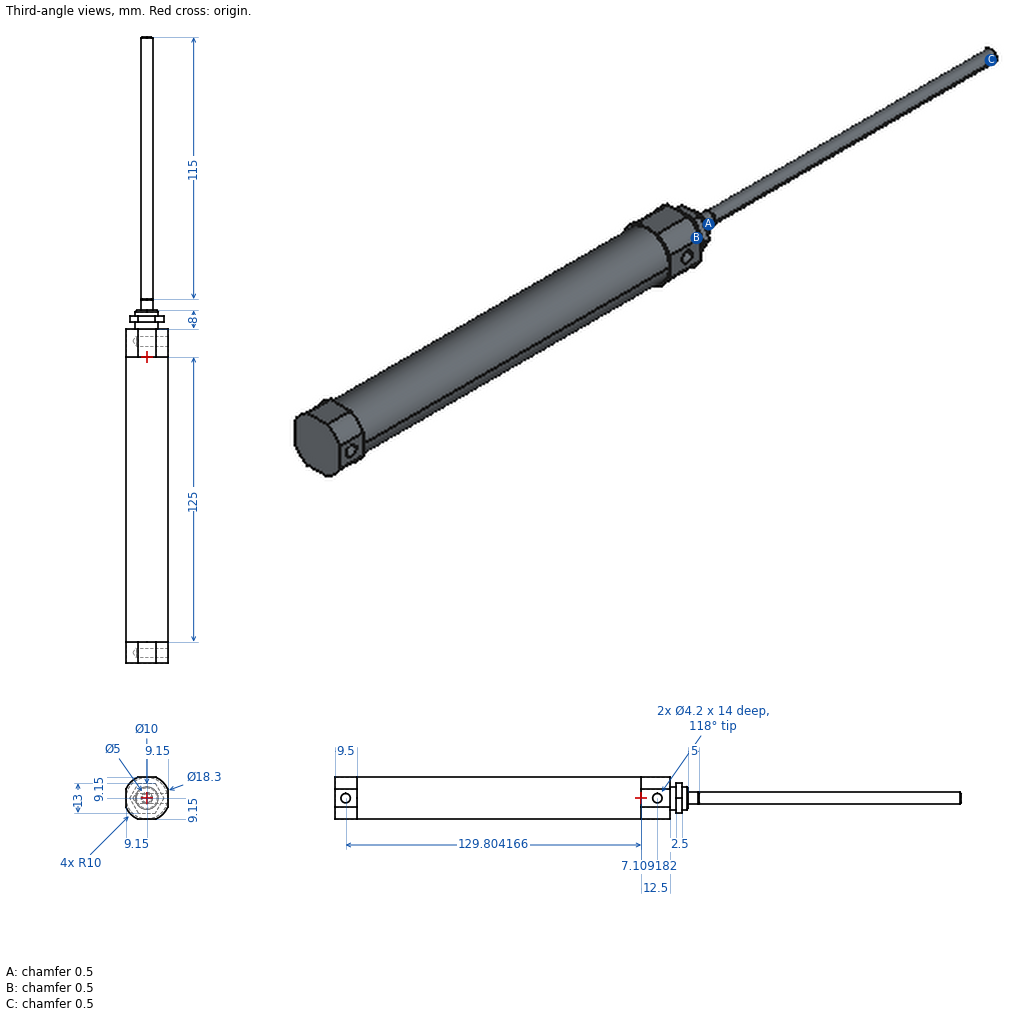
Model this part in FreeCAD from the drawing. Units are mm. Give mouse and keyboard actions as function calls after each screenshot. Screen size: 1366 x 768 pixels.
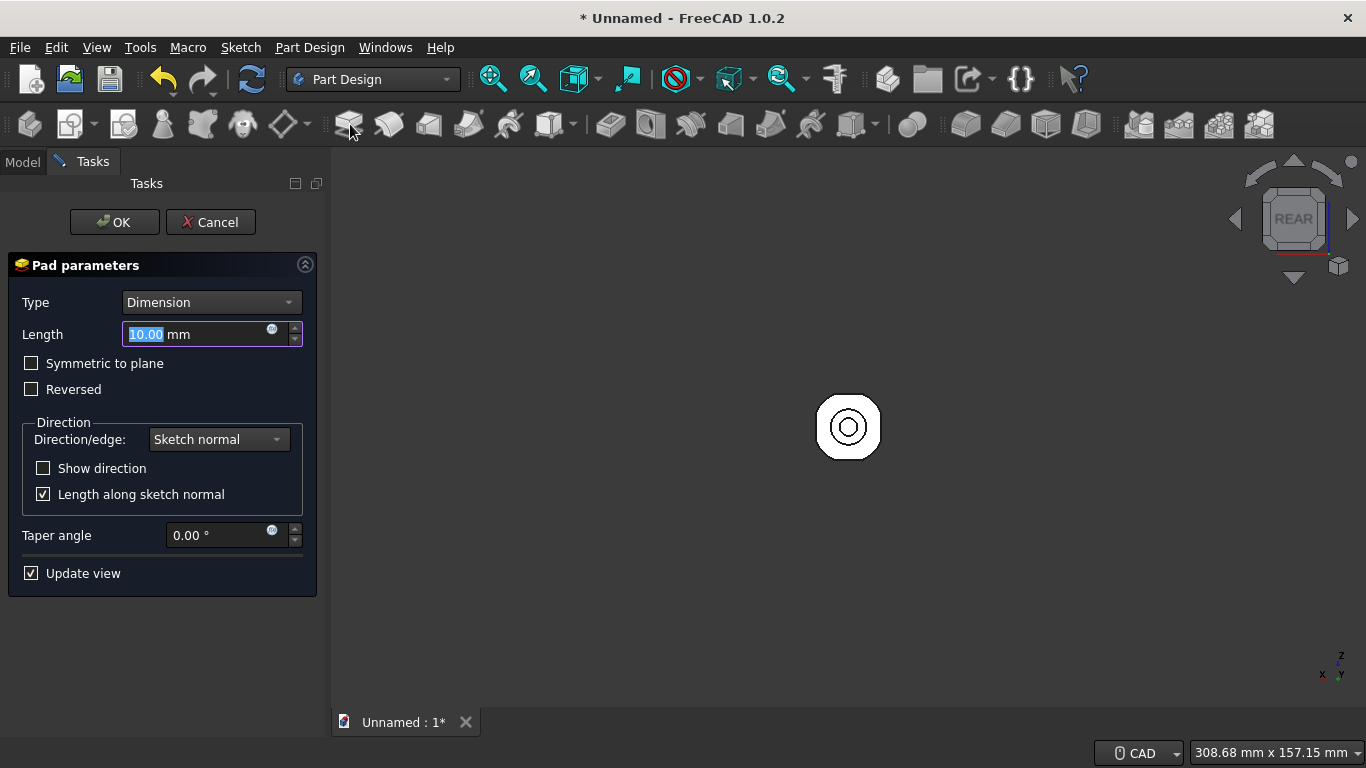
text(5)
key(Tab)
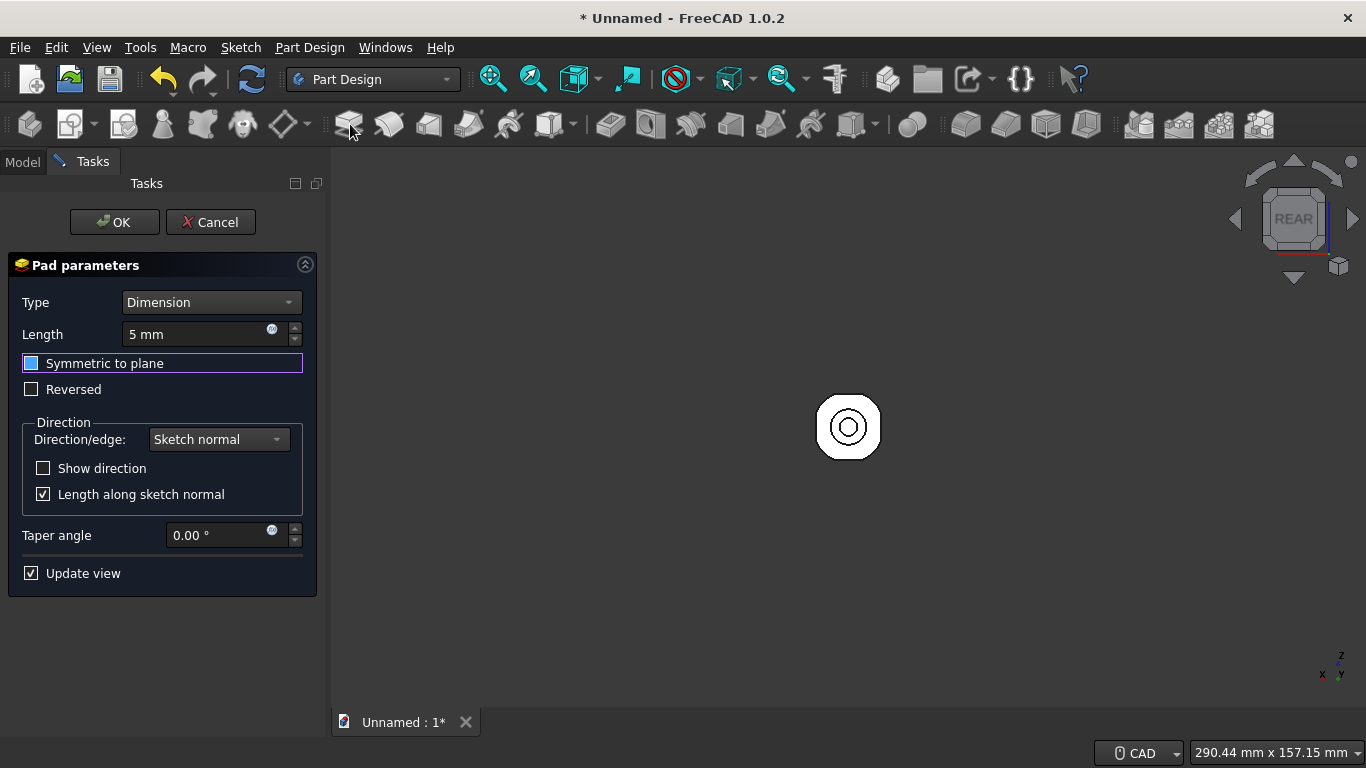
click(115, 222)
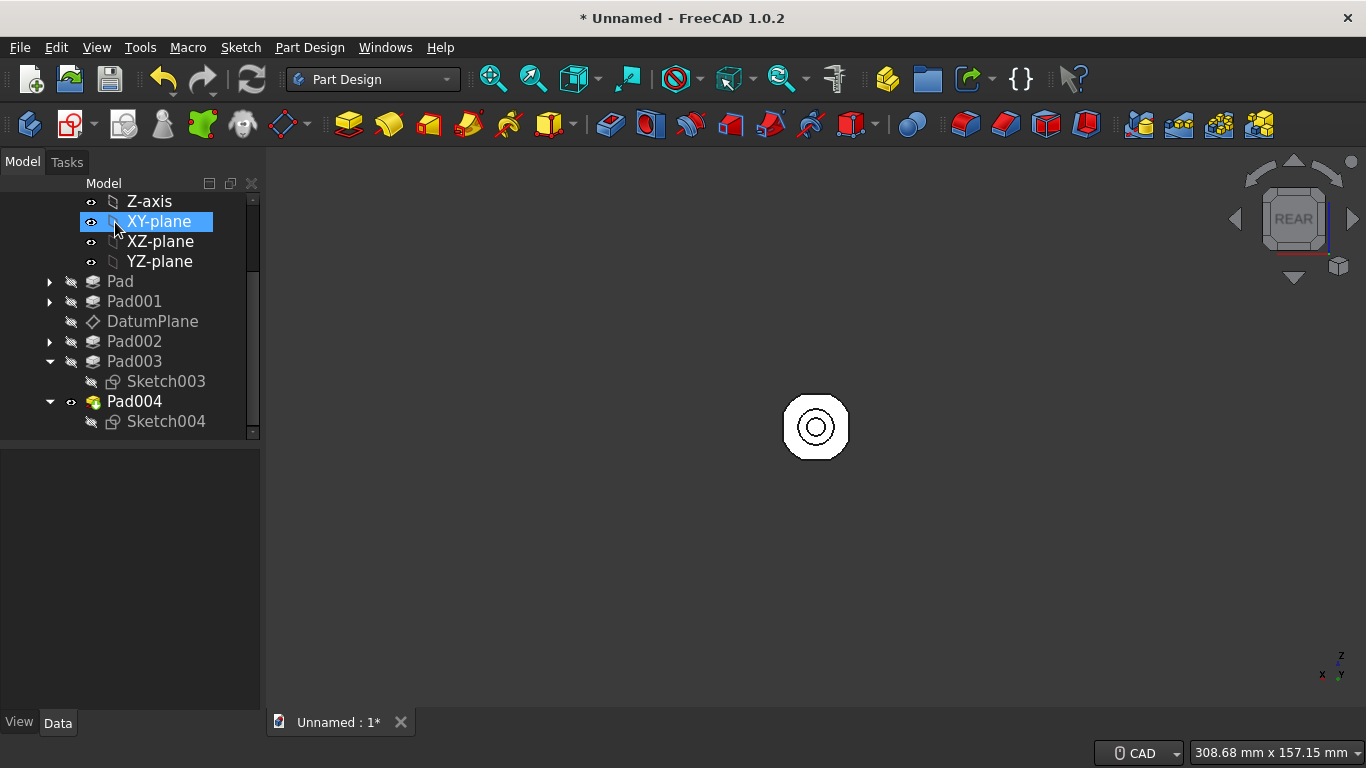
key(v)
key(f)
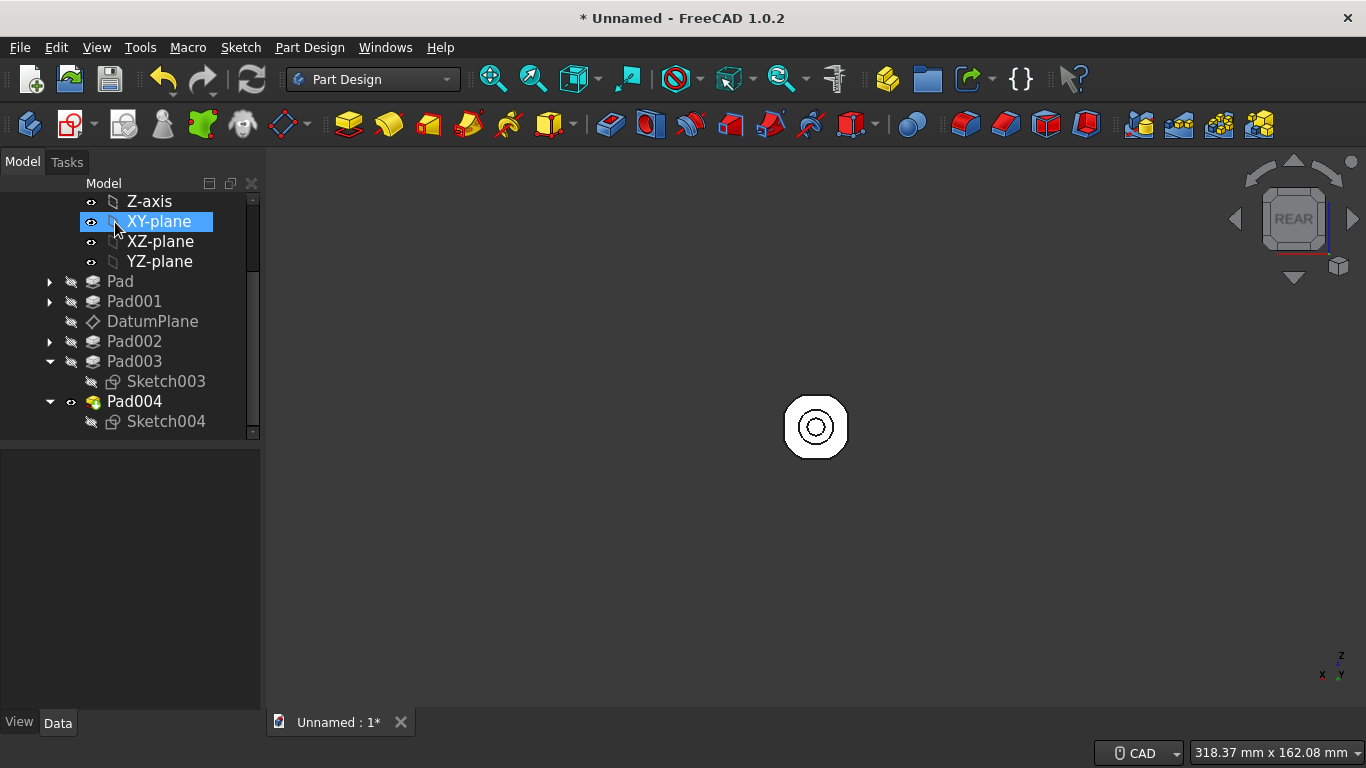
click(825, 426)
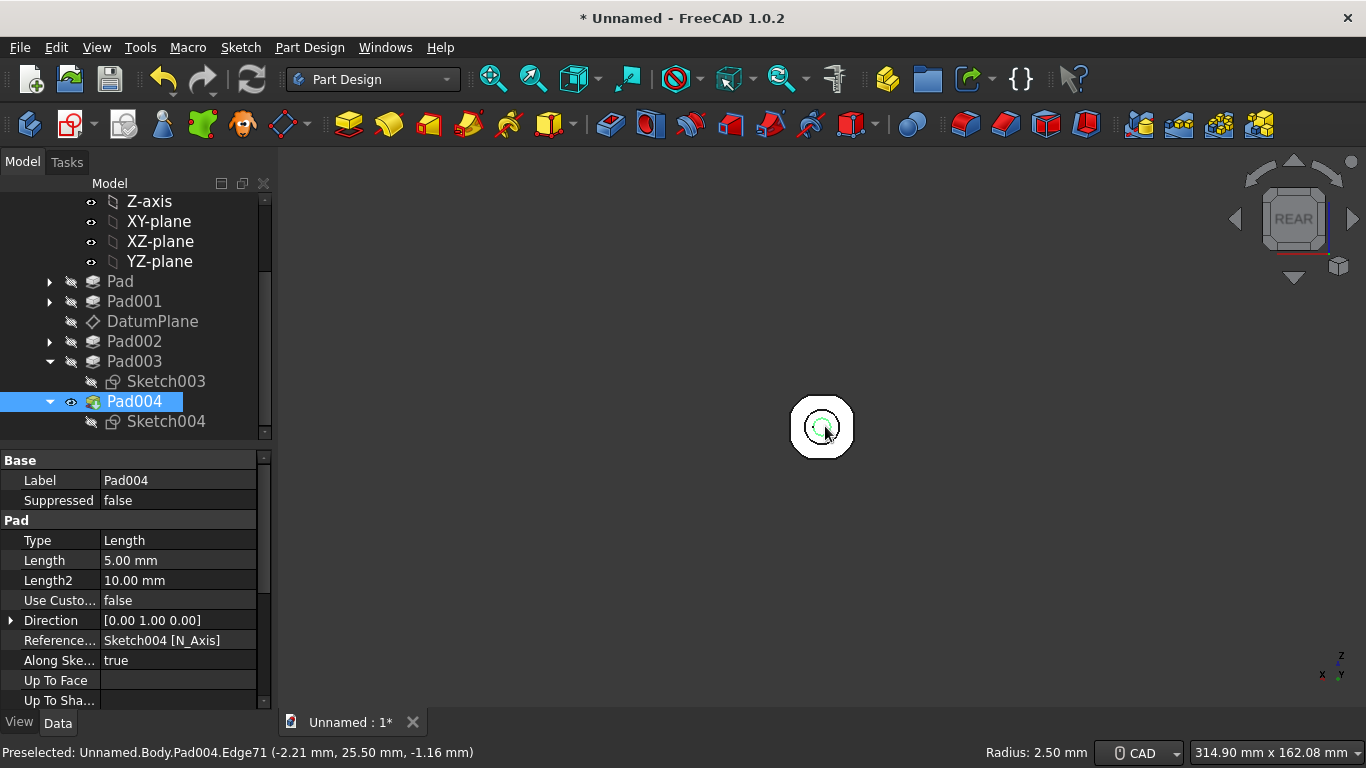
click(1006, 124)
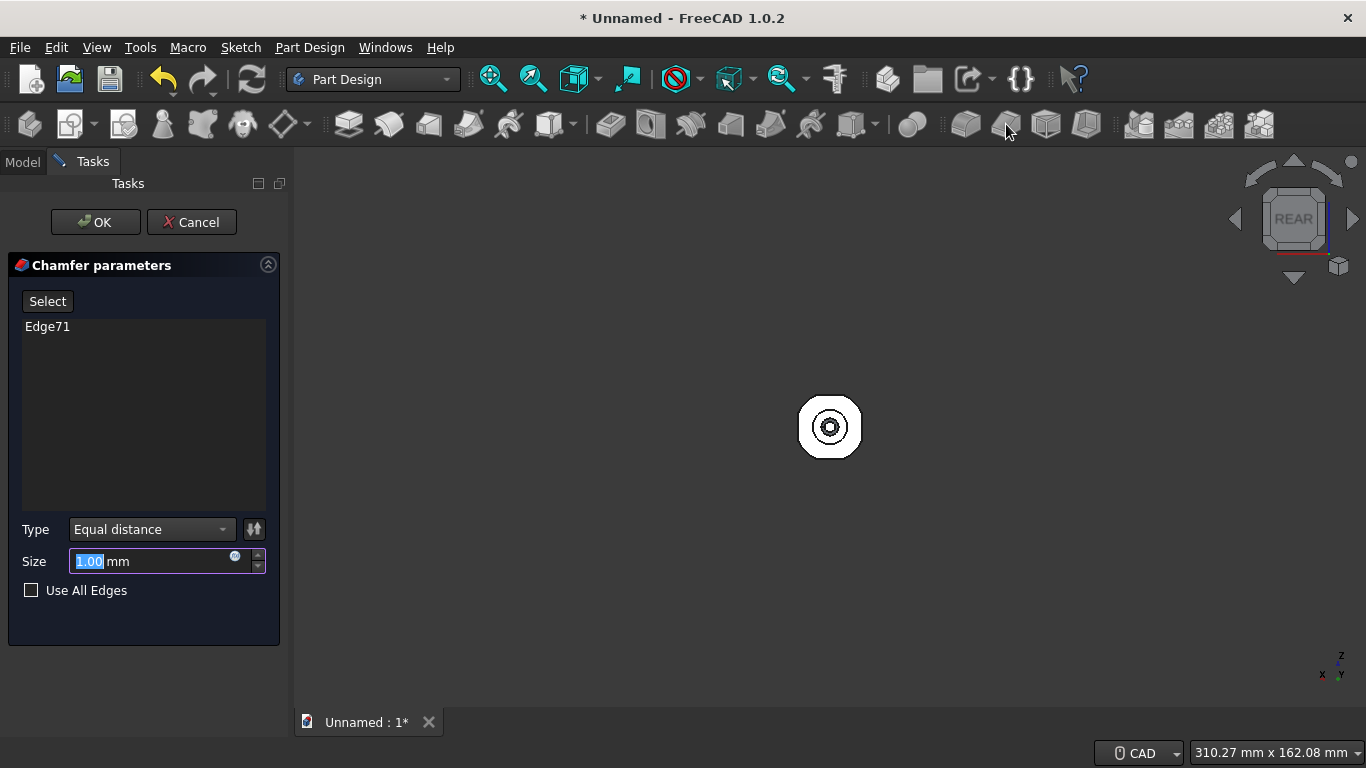
text(0.5)
key(Tab)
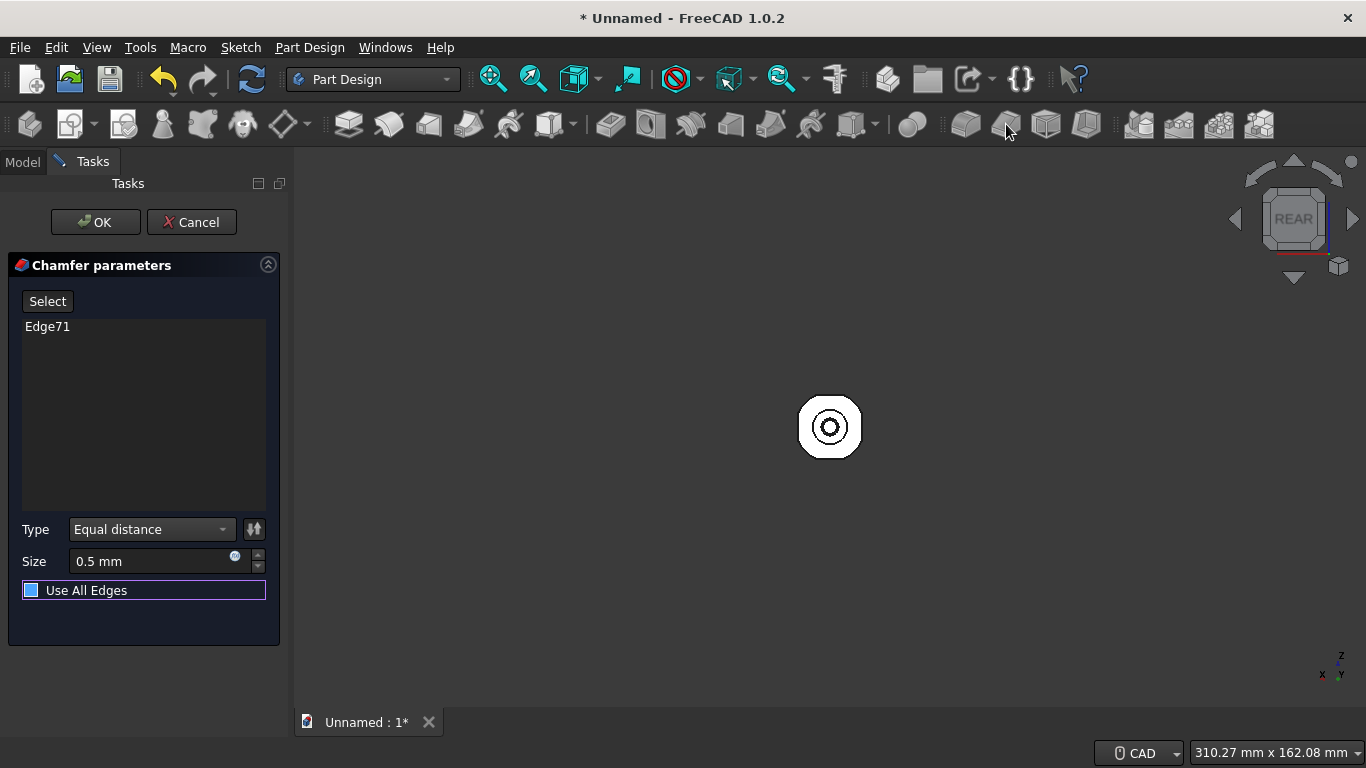
click(96, 222)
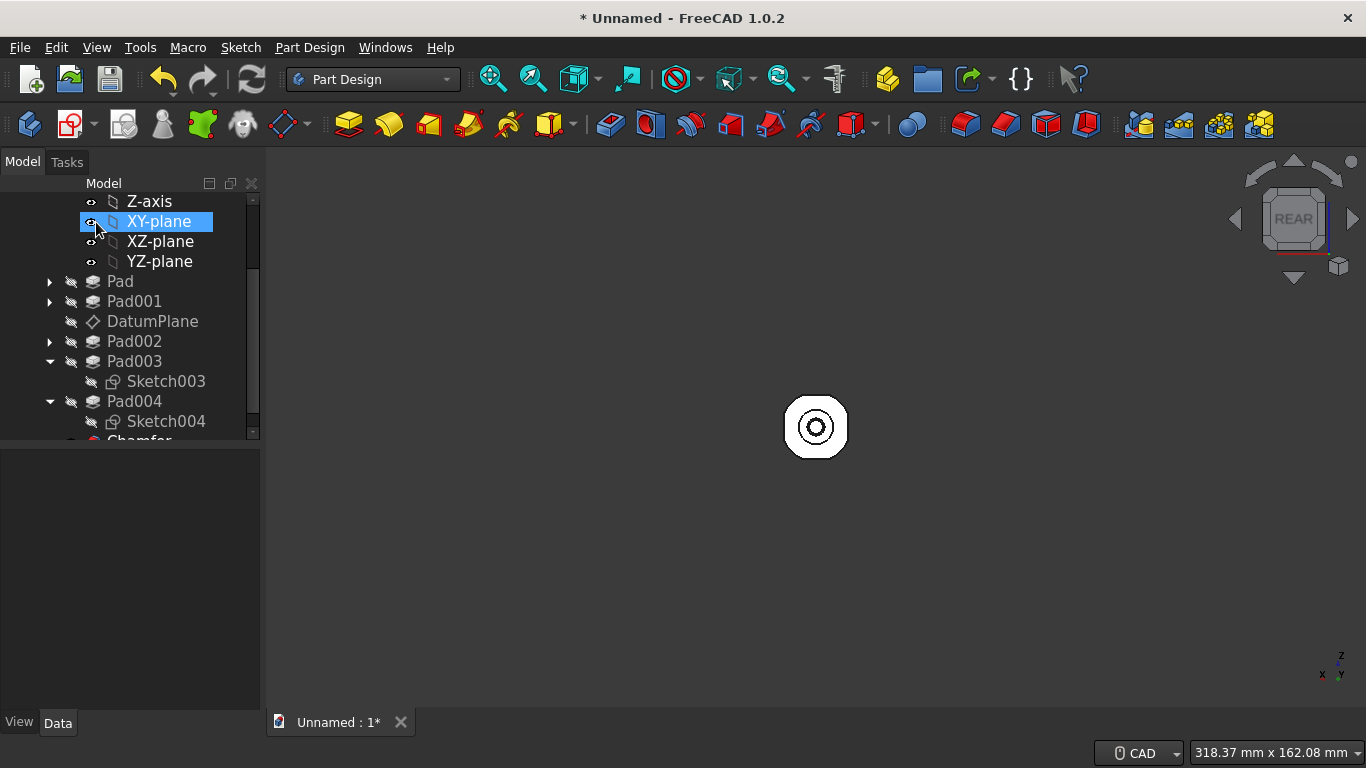
key(v)
key(f)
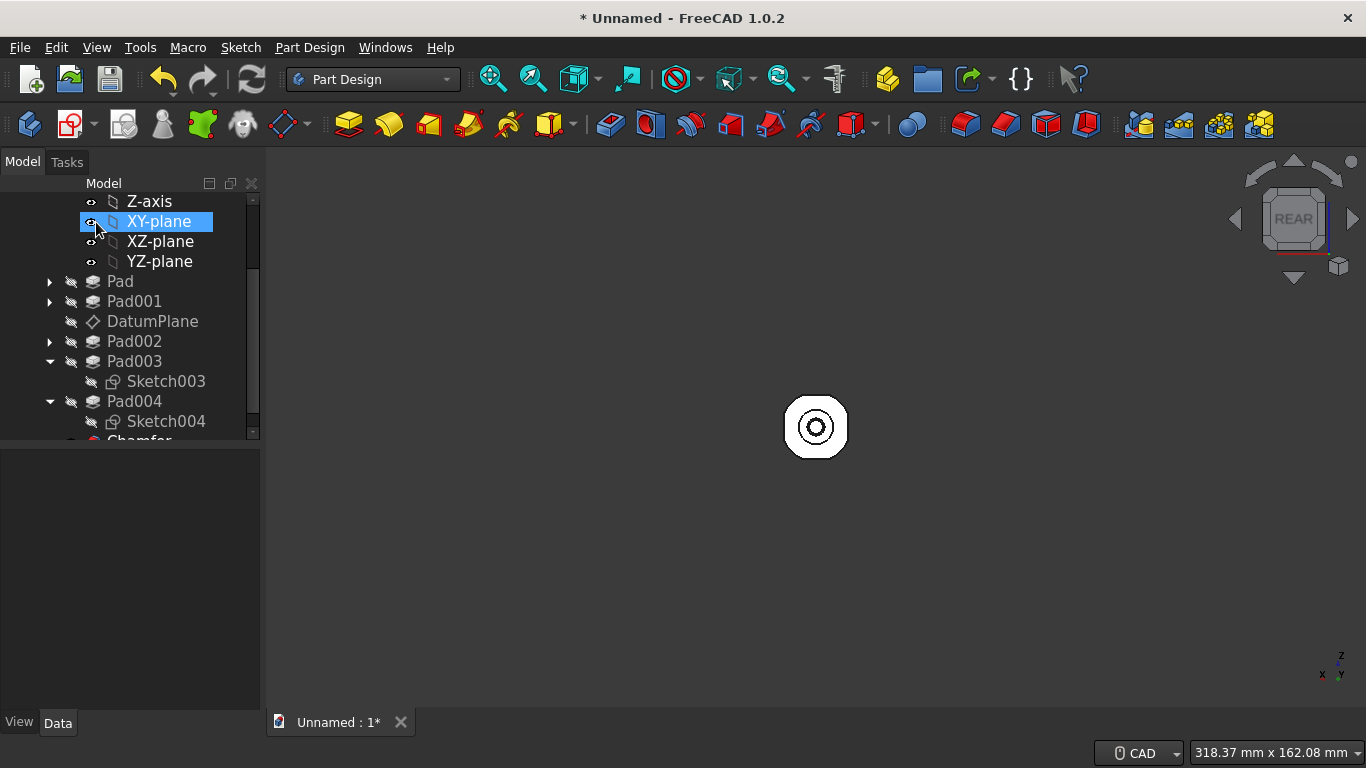
scroll(816, 426, up, 3)